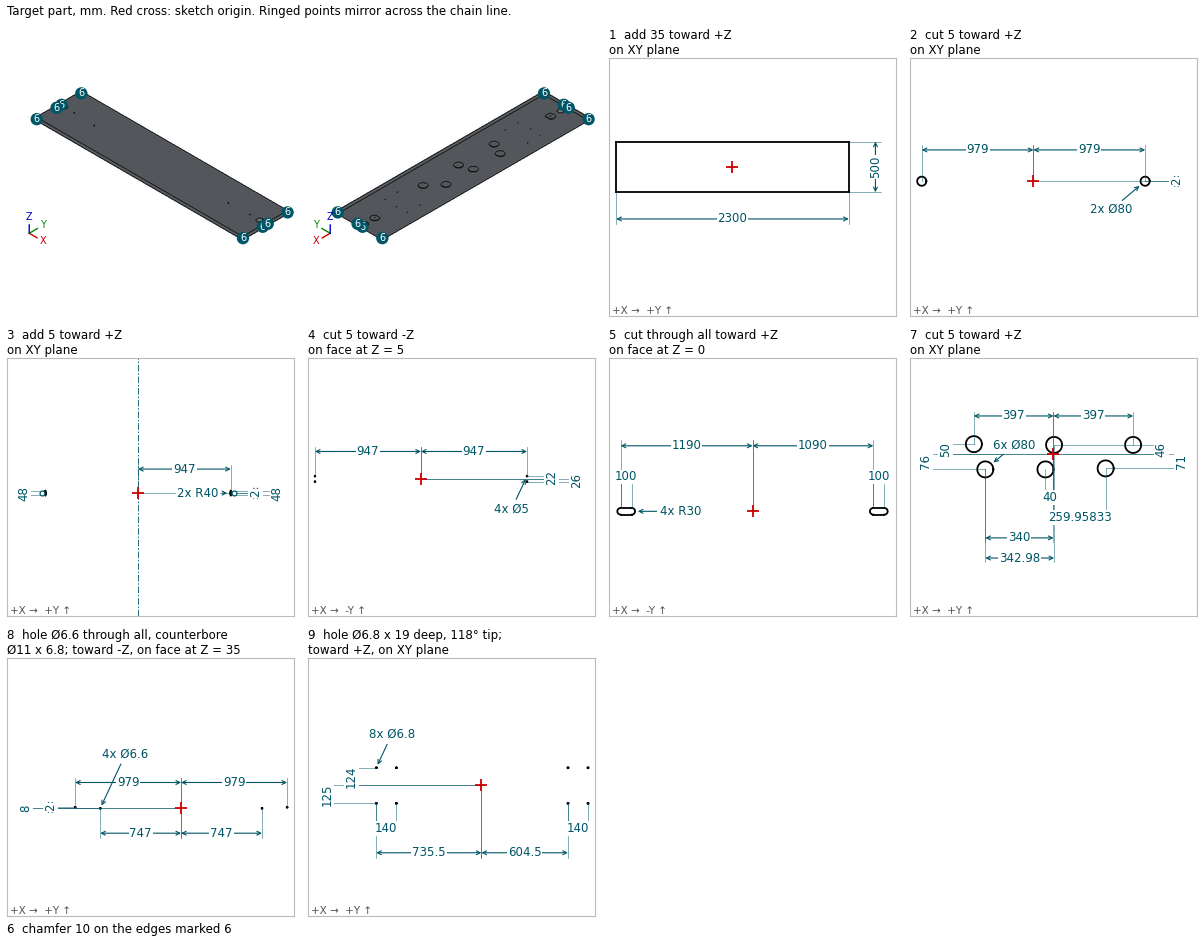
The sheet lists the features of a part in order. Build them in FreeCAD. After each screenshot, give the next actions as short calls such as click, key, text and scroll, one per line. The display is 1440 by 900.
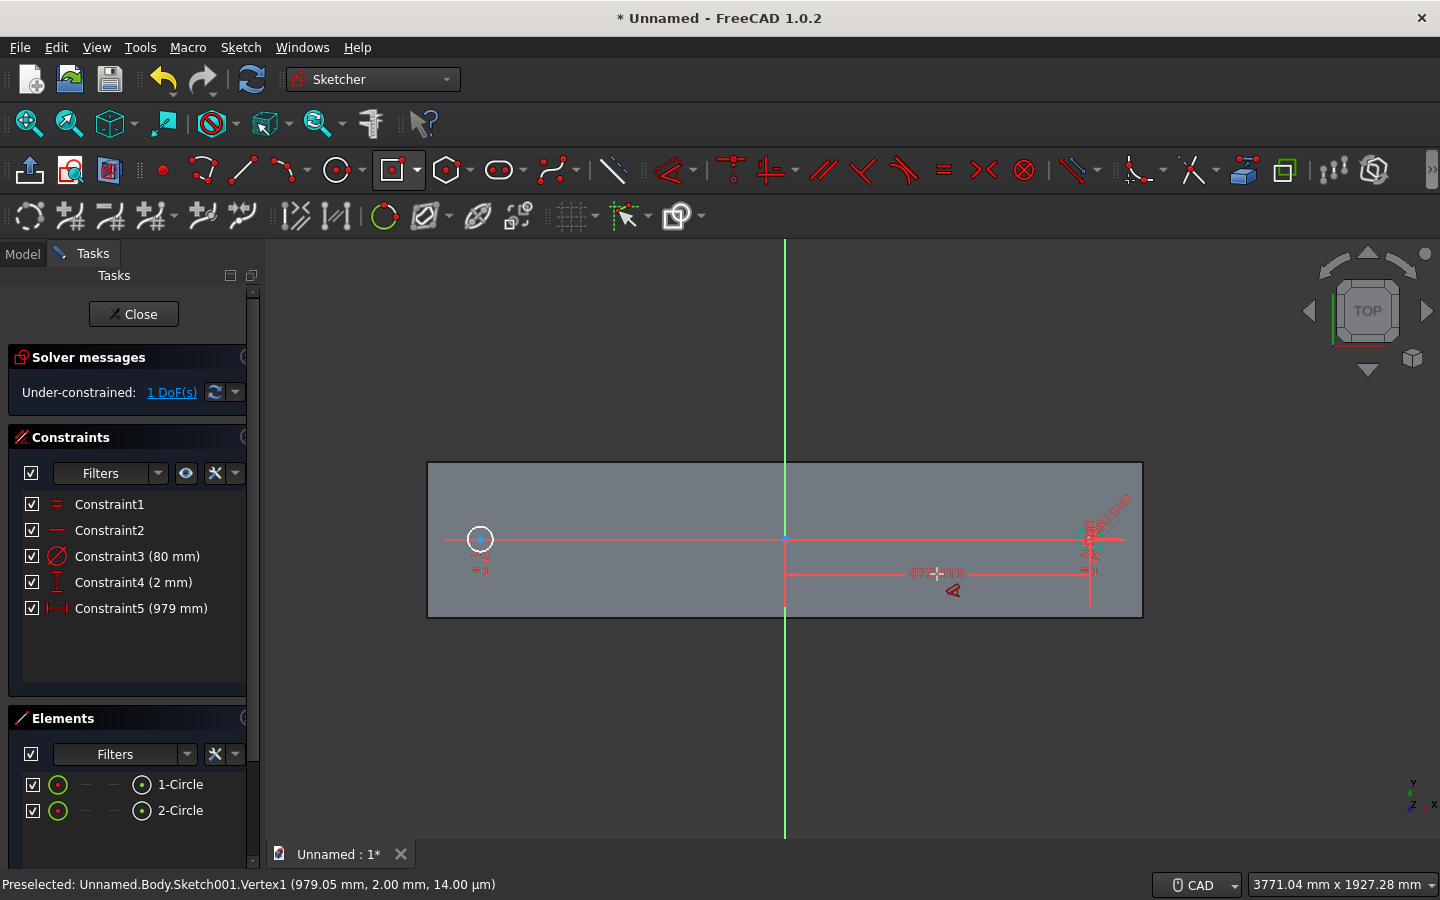
click(480, 539)
click(633, 574)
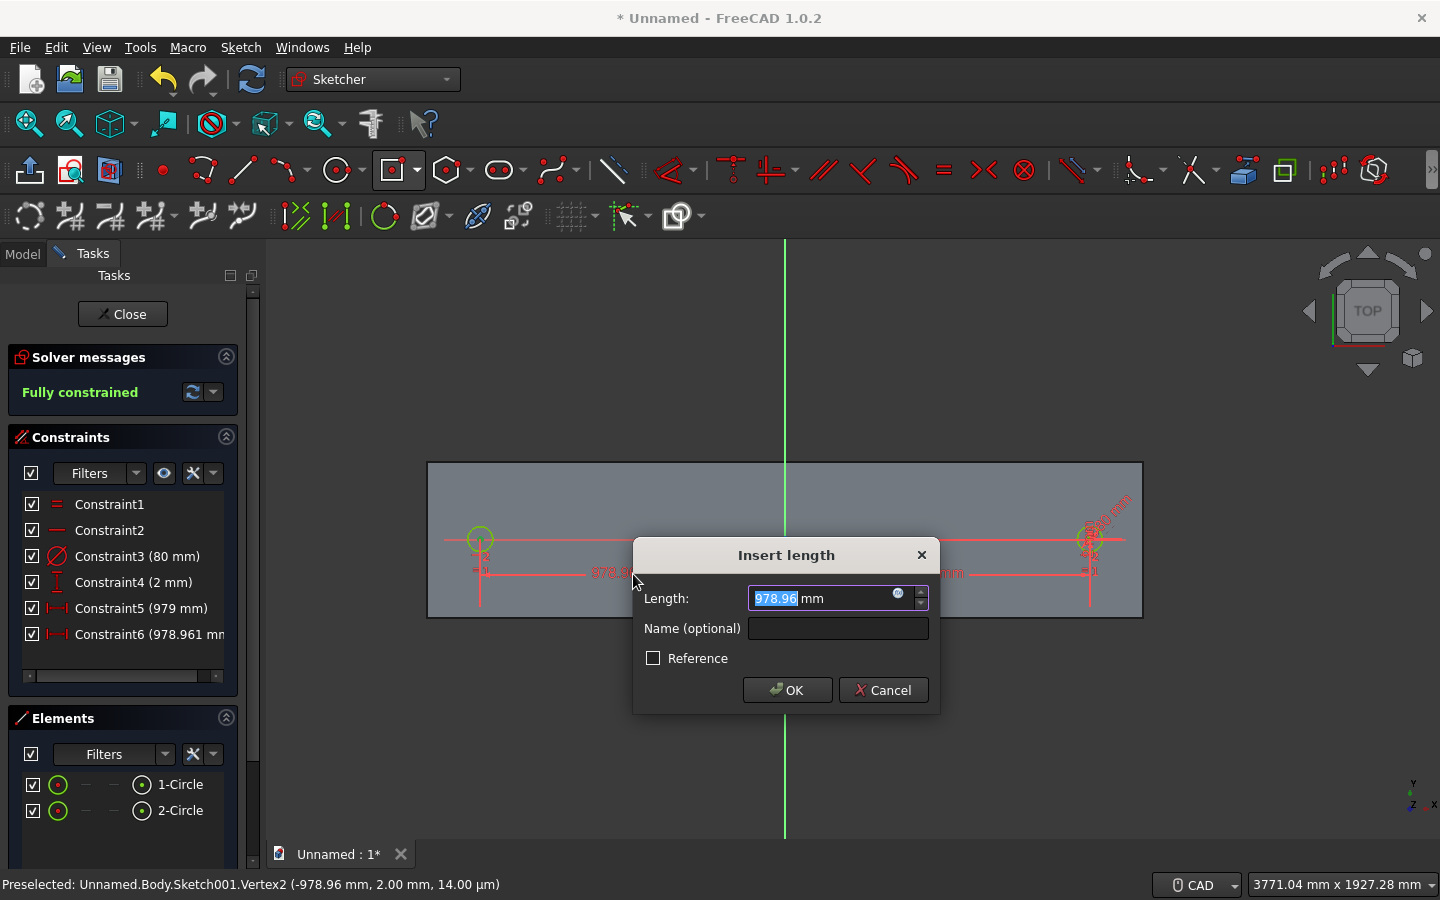
text(979)
key(Return)
key(Escape)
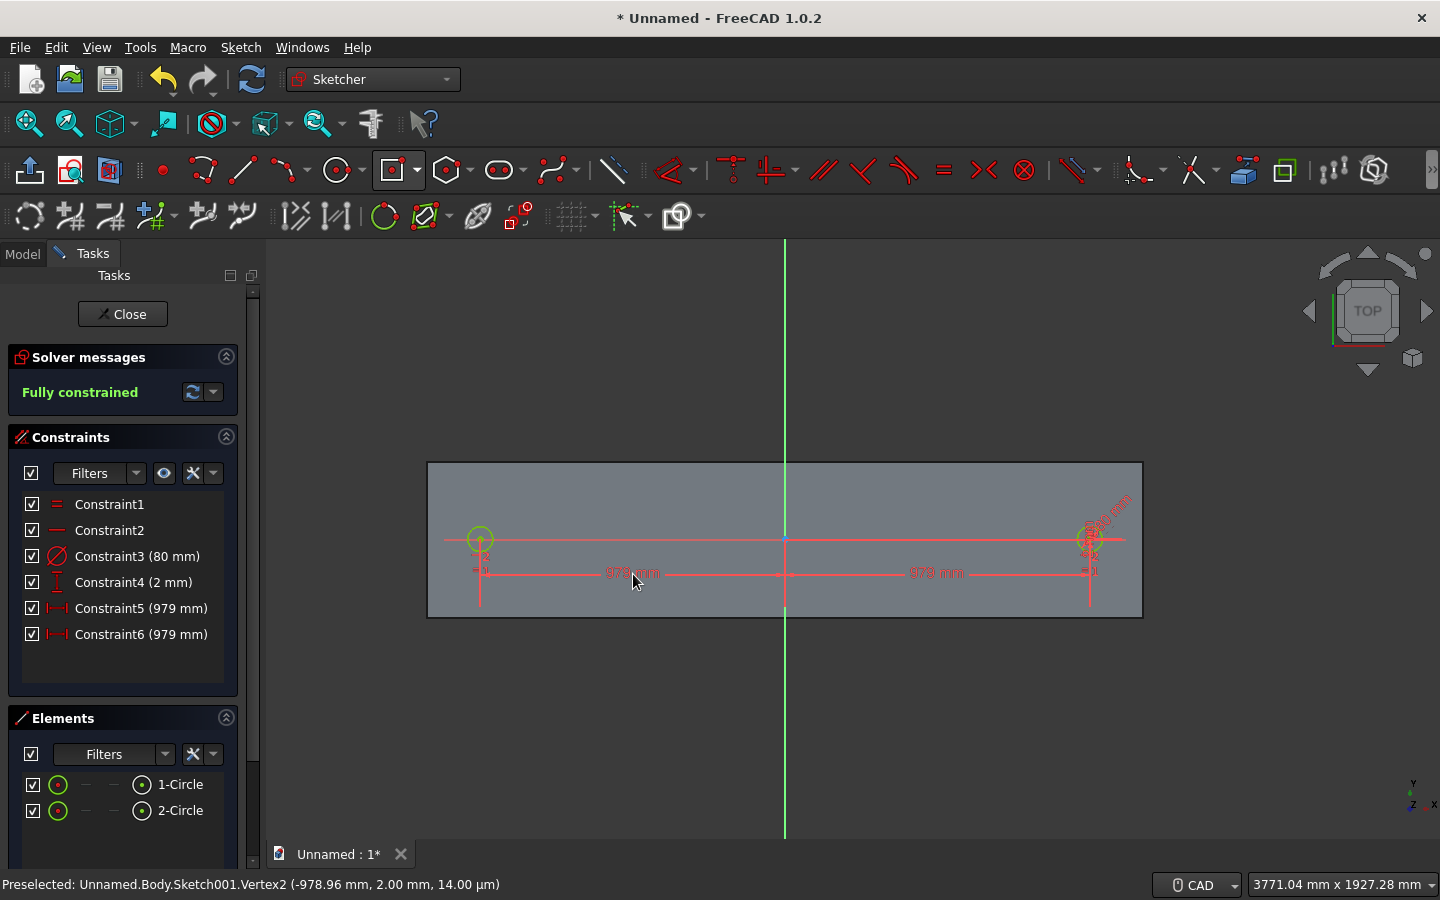
click(123, 314)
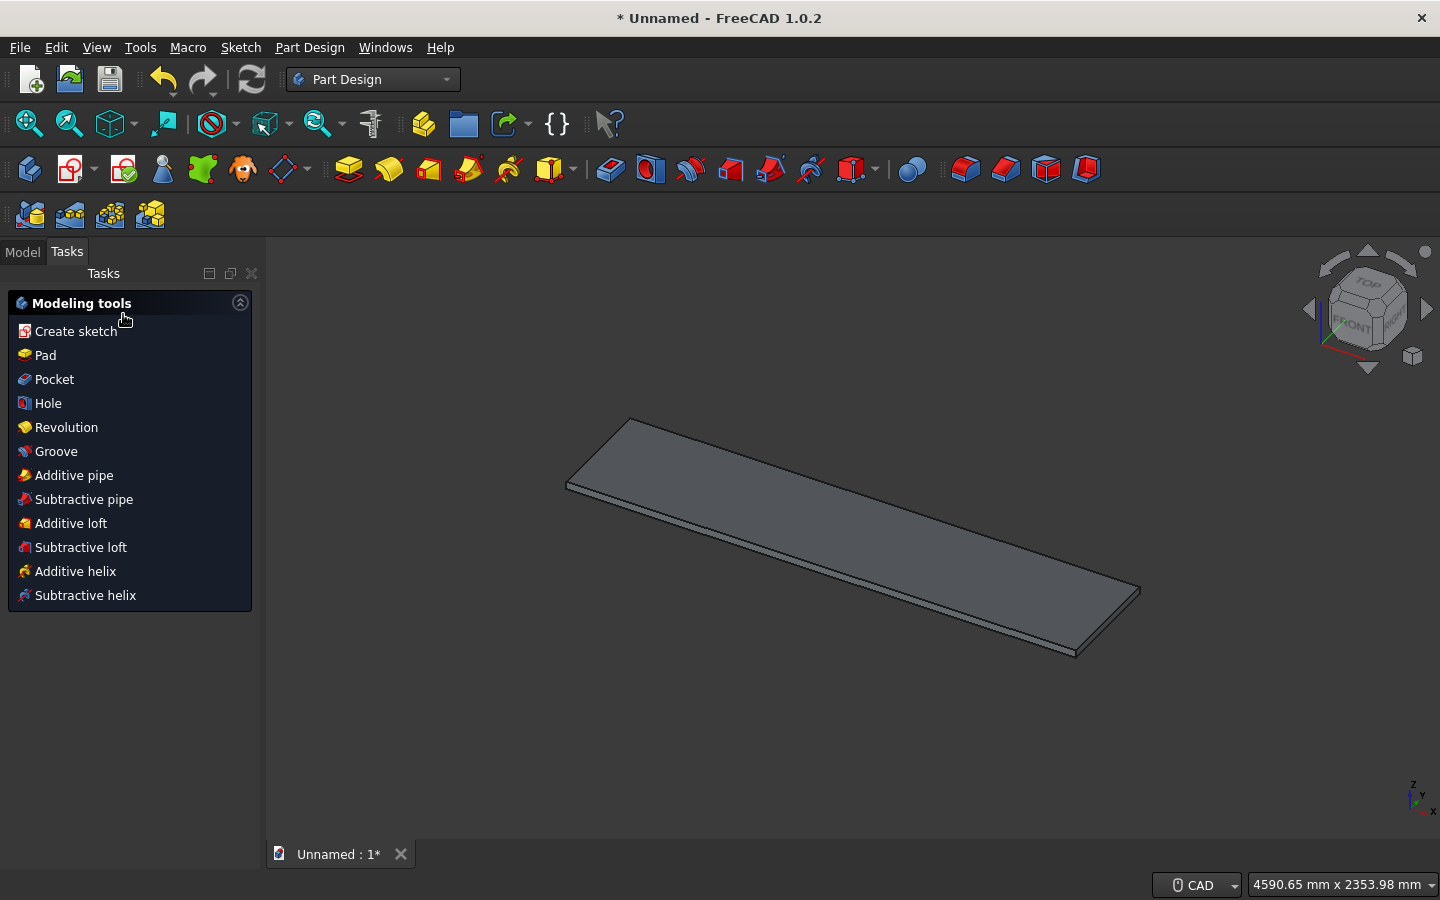
click(612, 170)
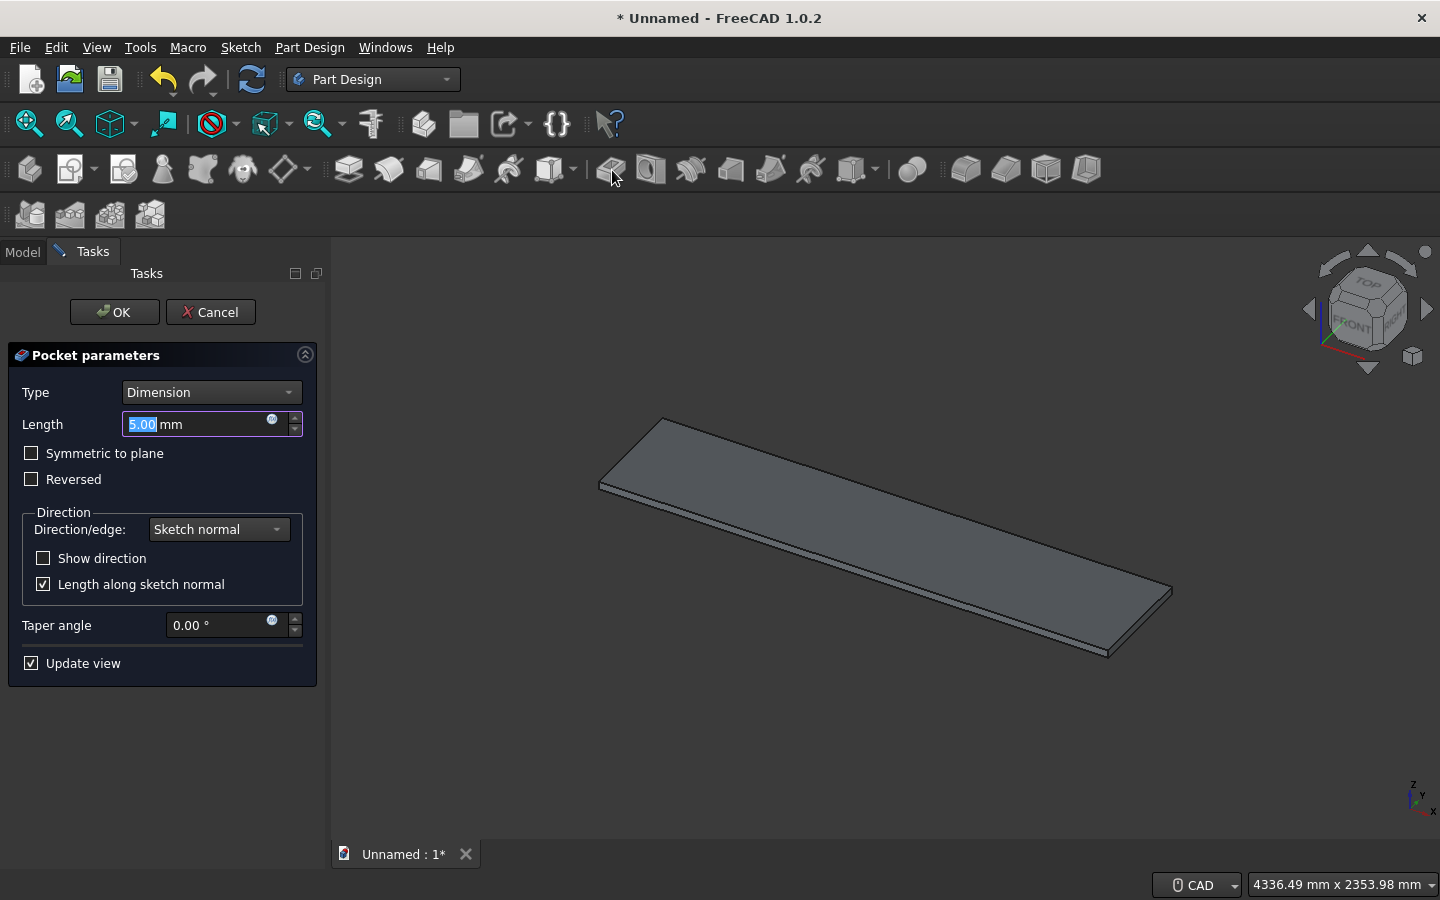
text(5)
key(Tab)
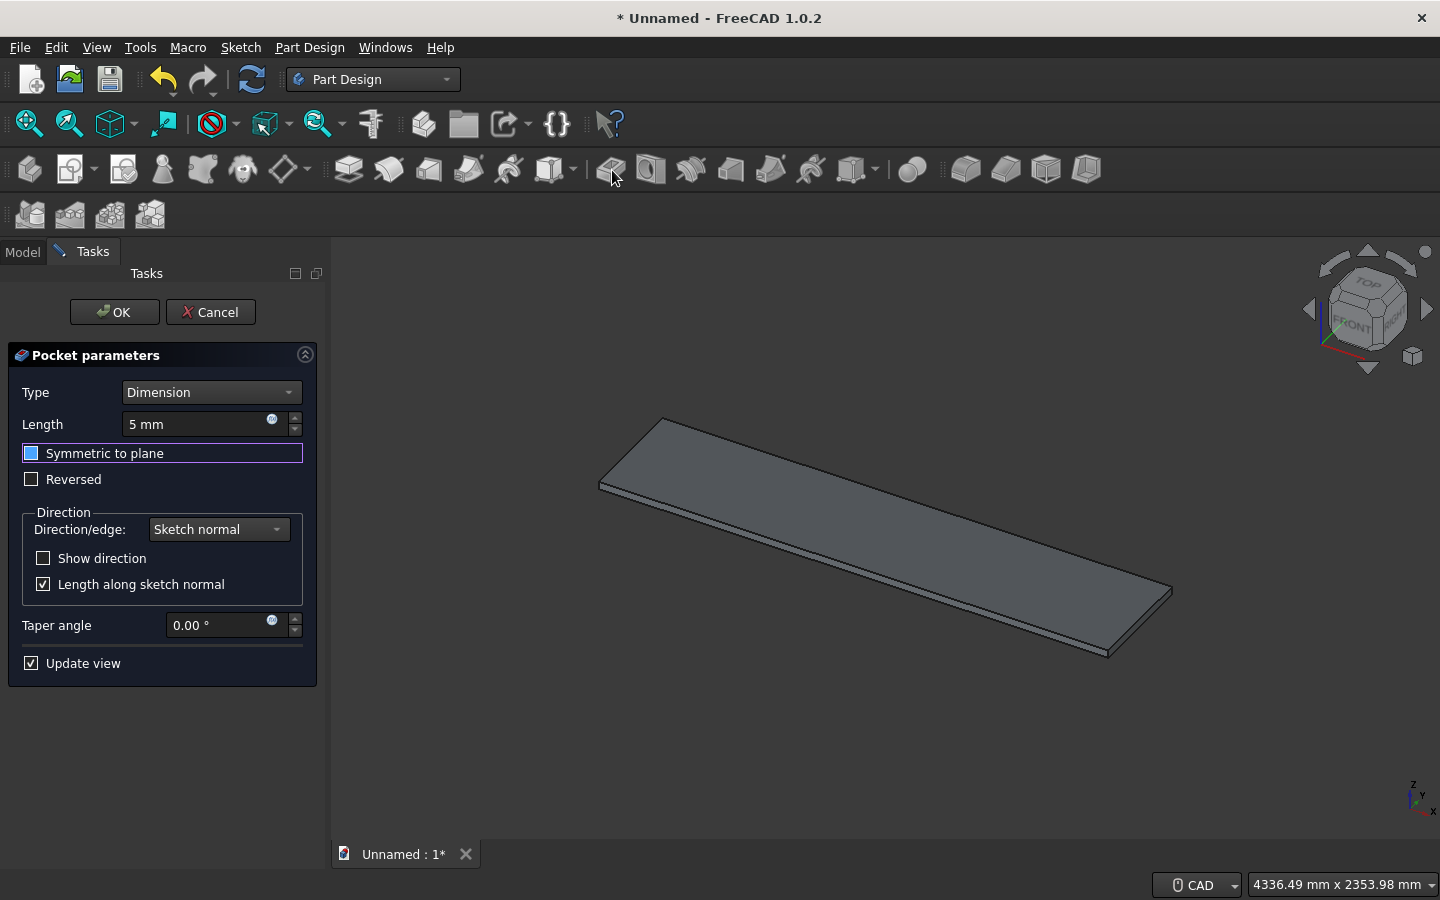
click(30, 479)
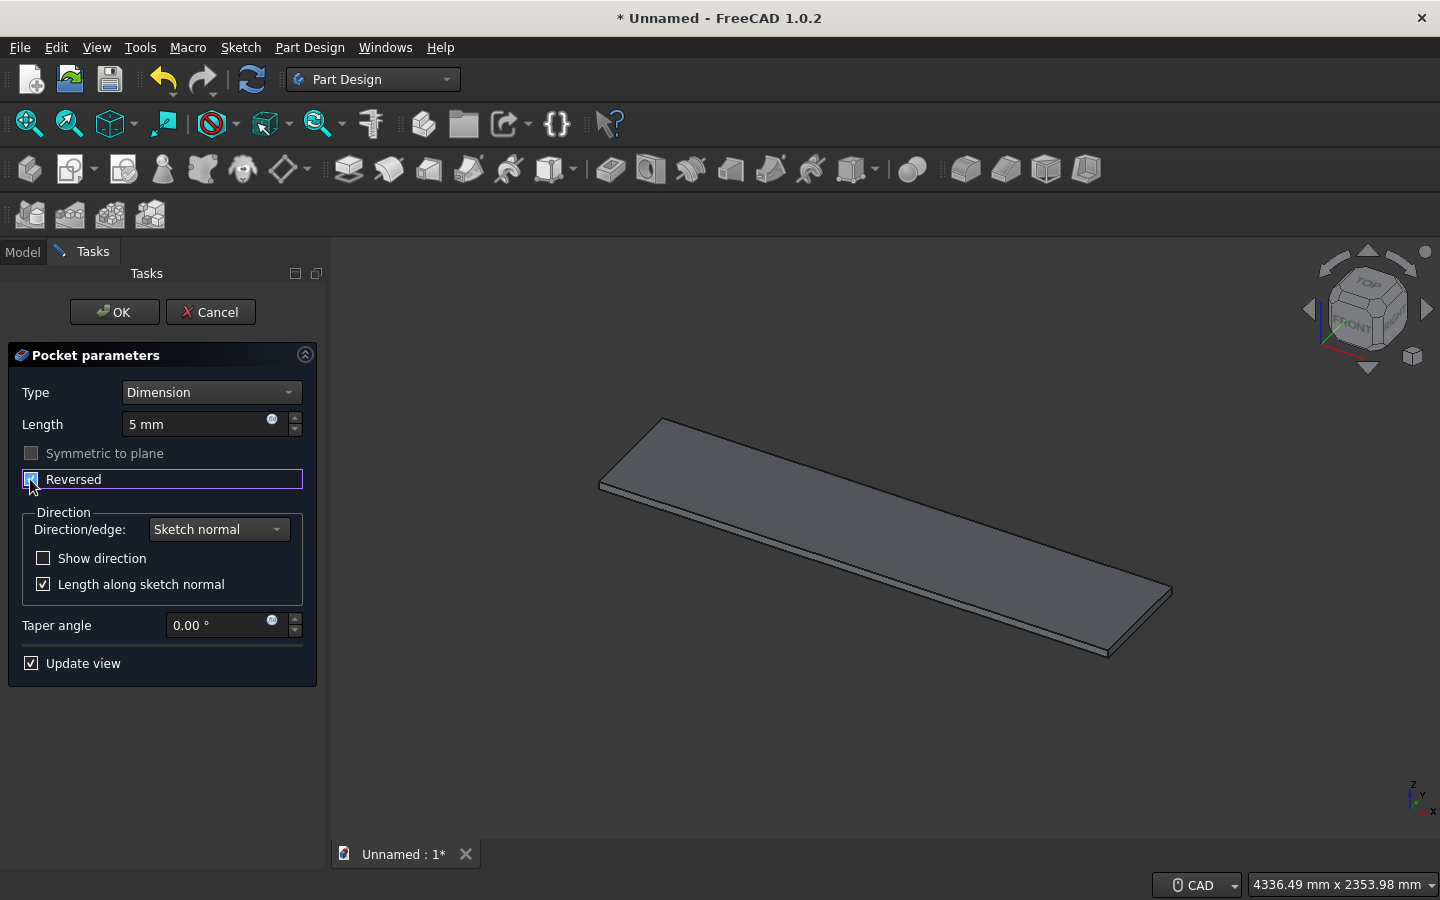
click(115, 312)